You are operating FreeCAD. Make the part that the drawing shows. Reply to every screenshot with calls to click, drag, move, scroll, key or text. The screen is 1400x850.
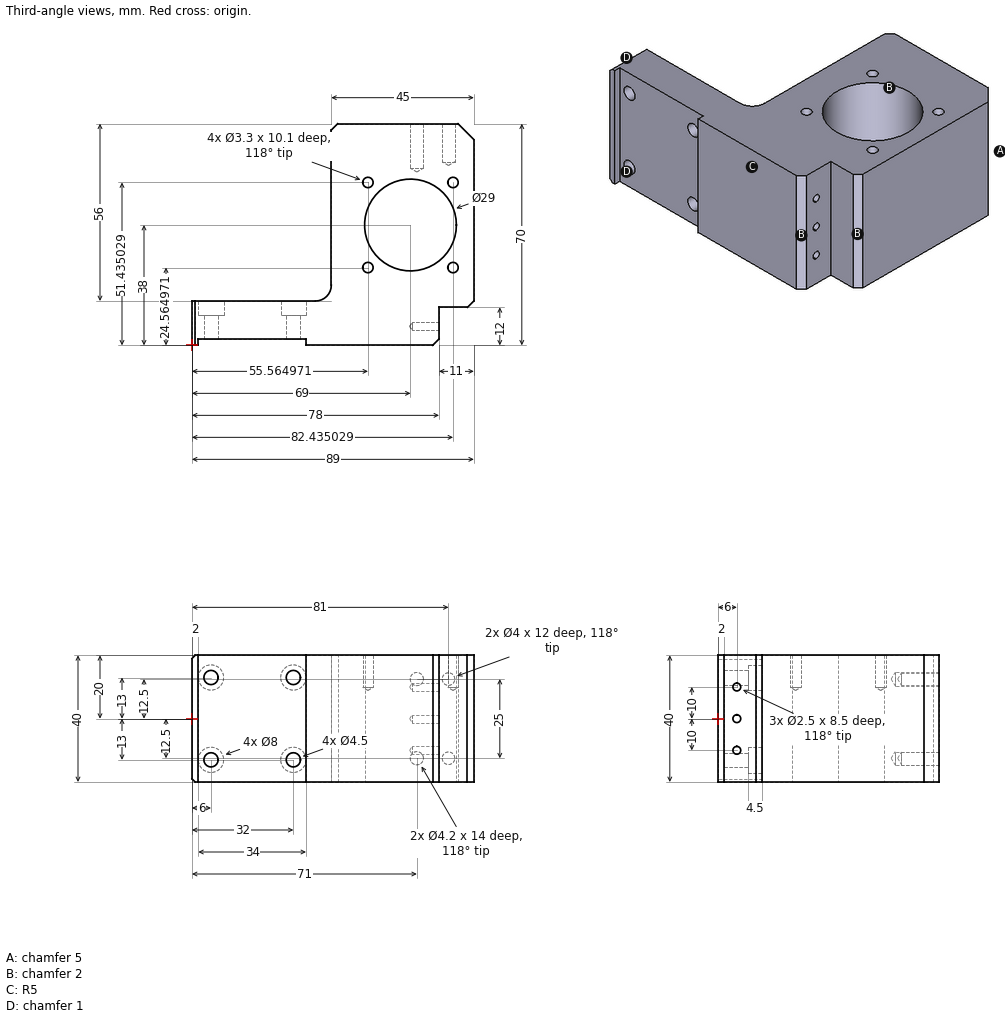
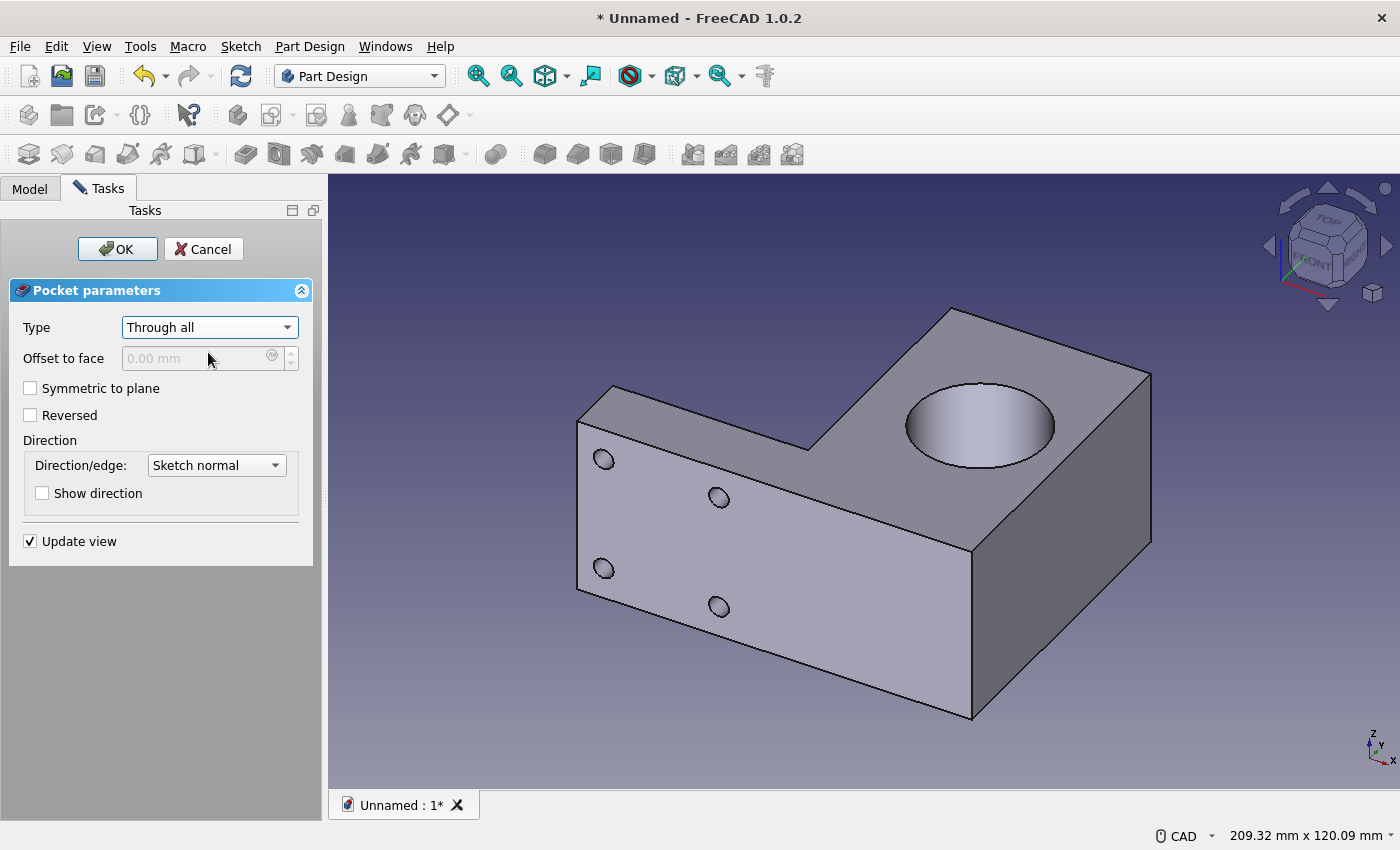
click(118, 249)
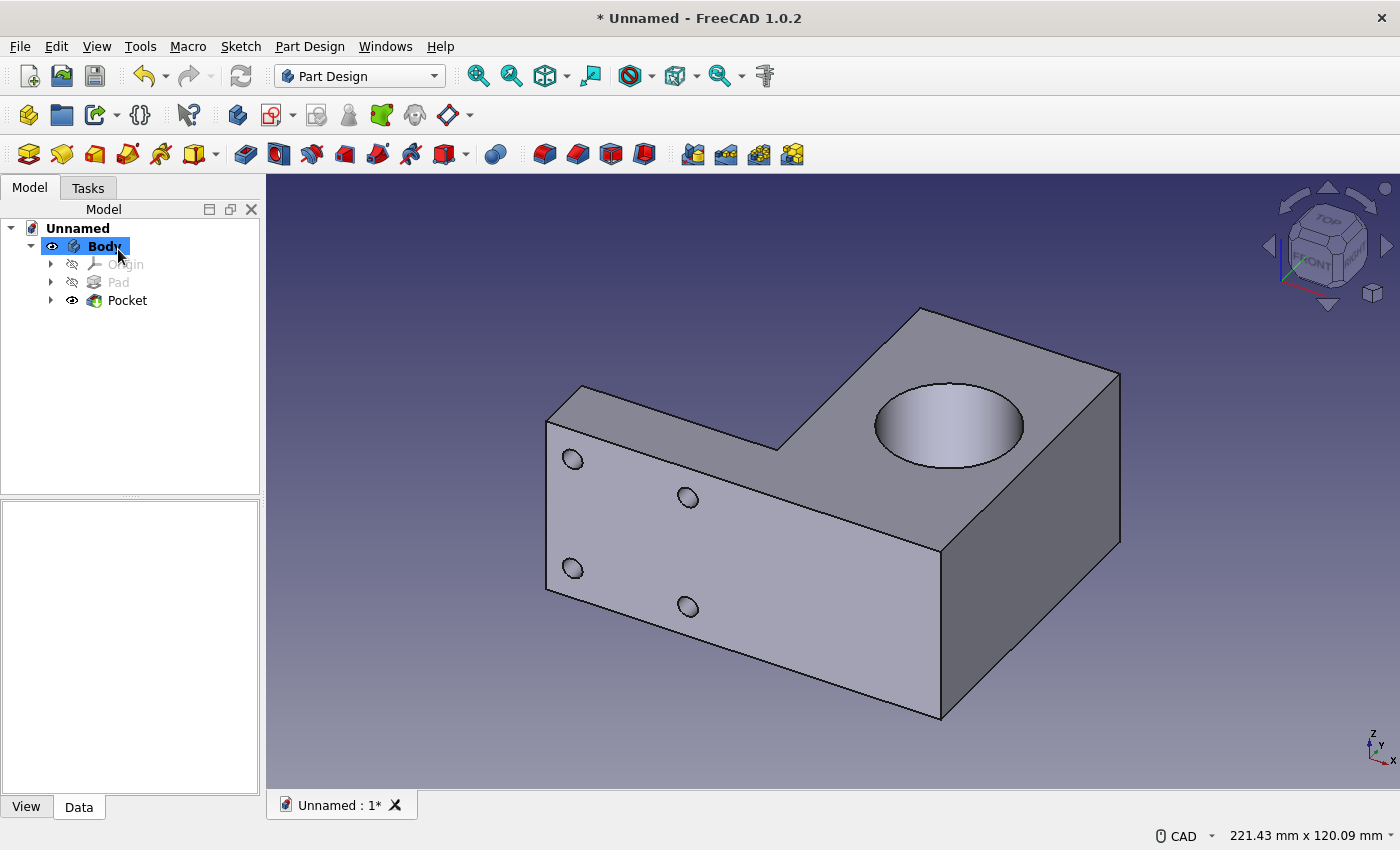
click(270, 116)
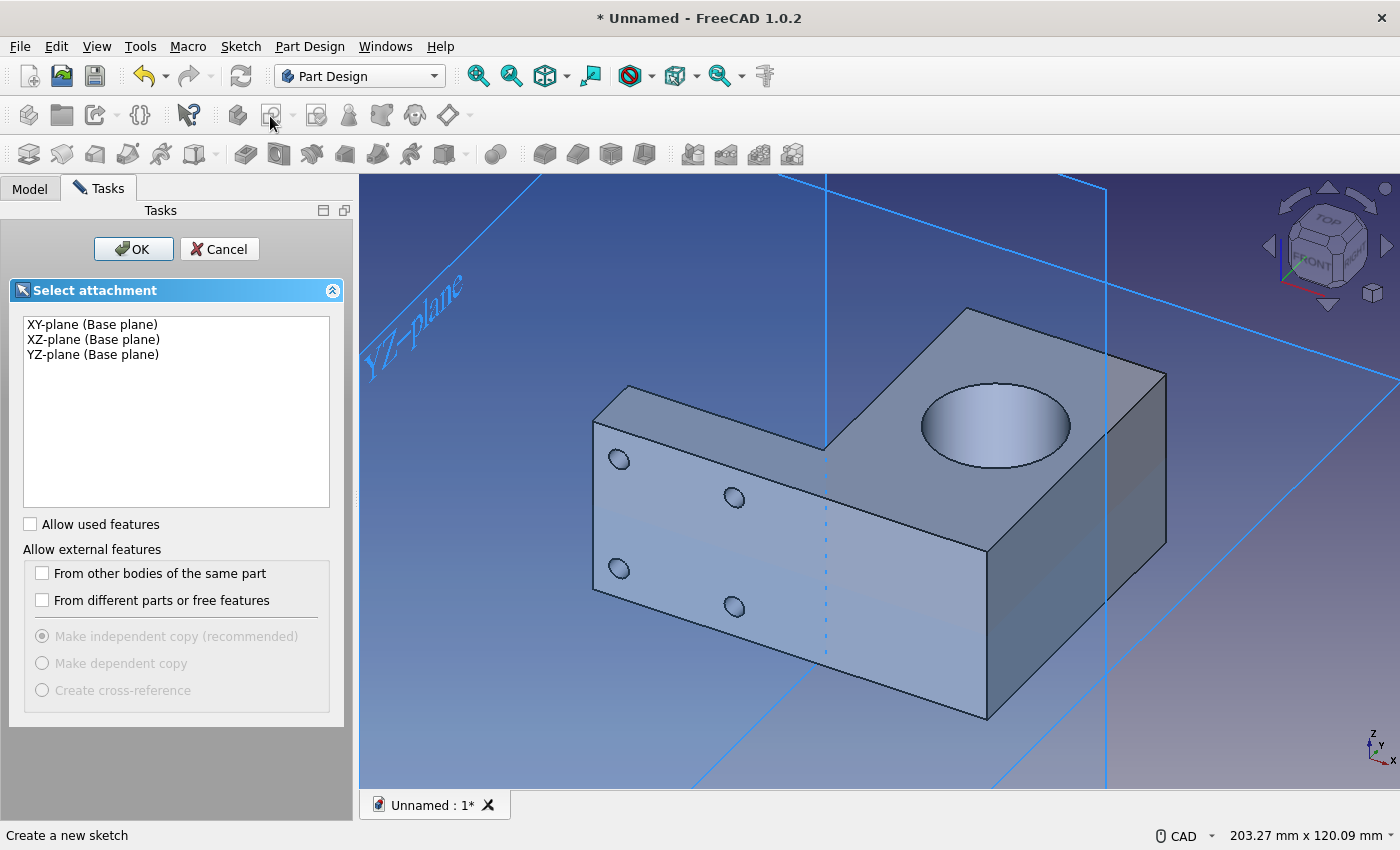
click(84, 340)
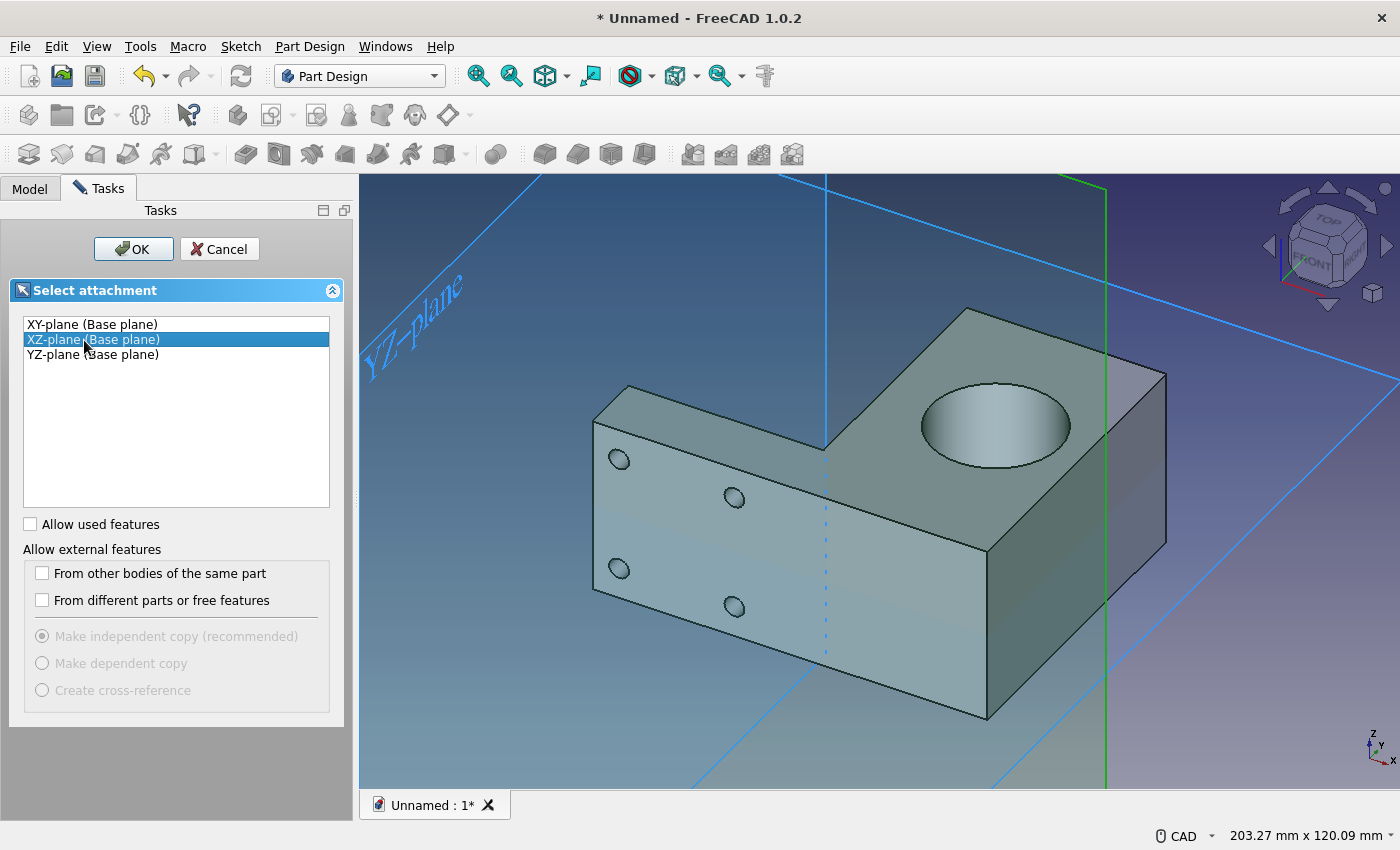
click(134, 249)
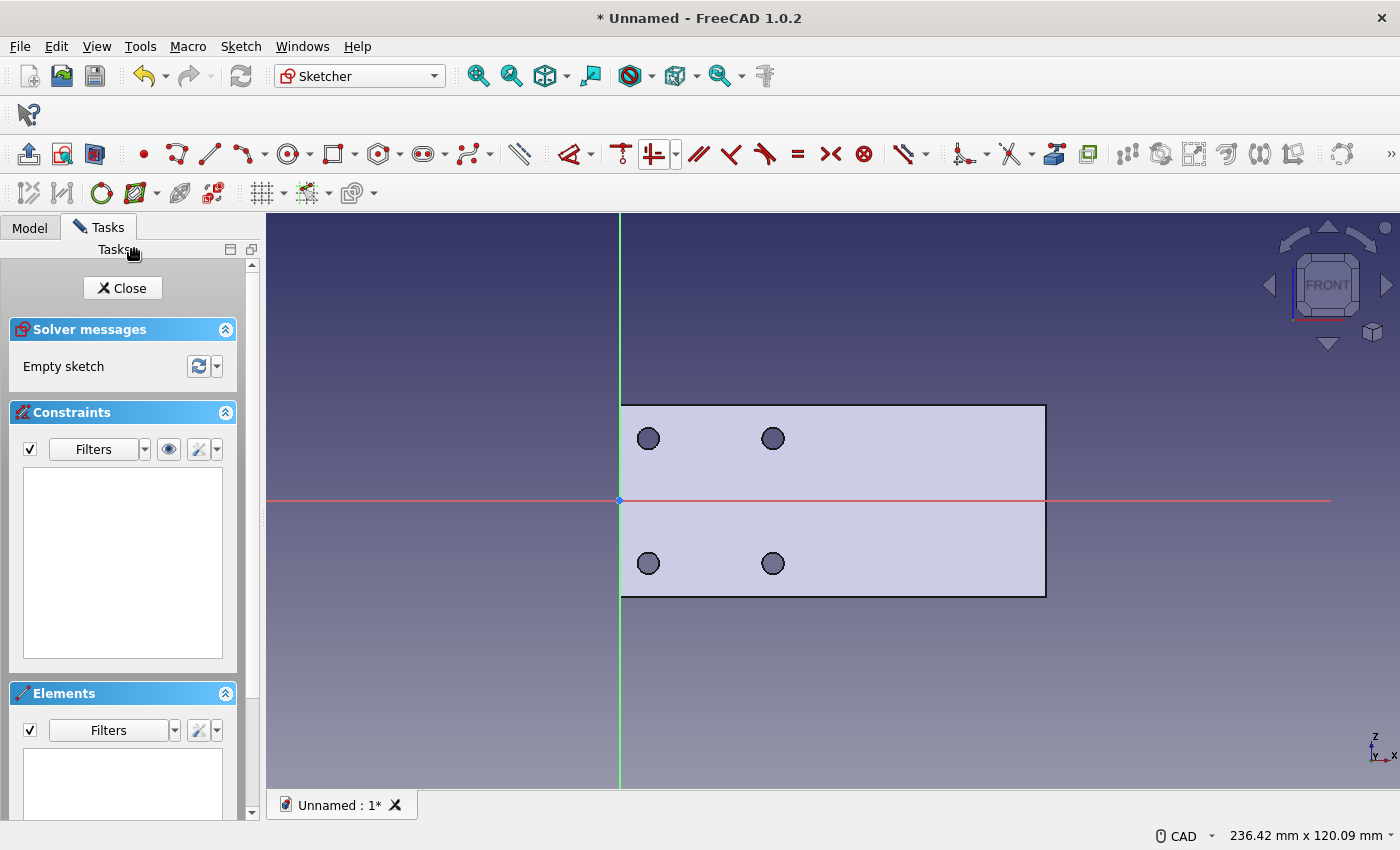
scroll(635, 501, up, 3)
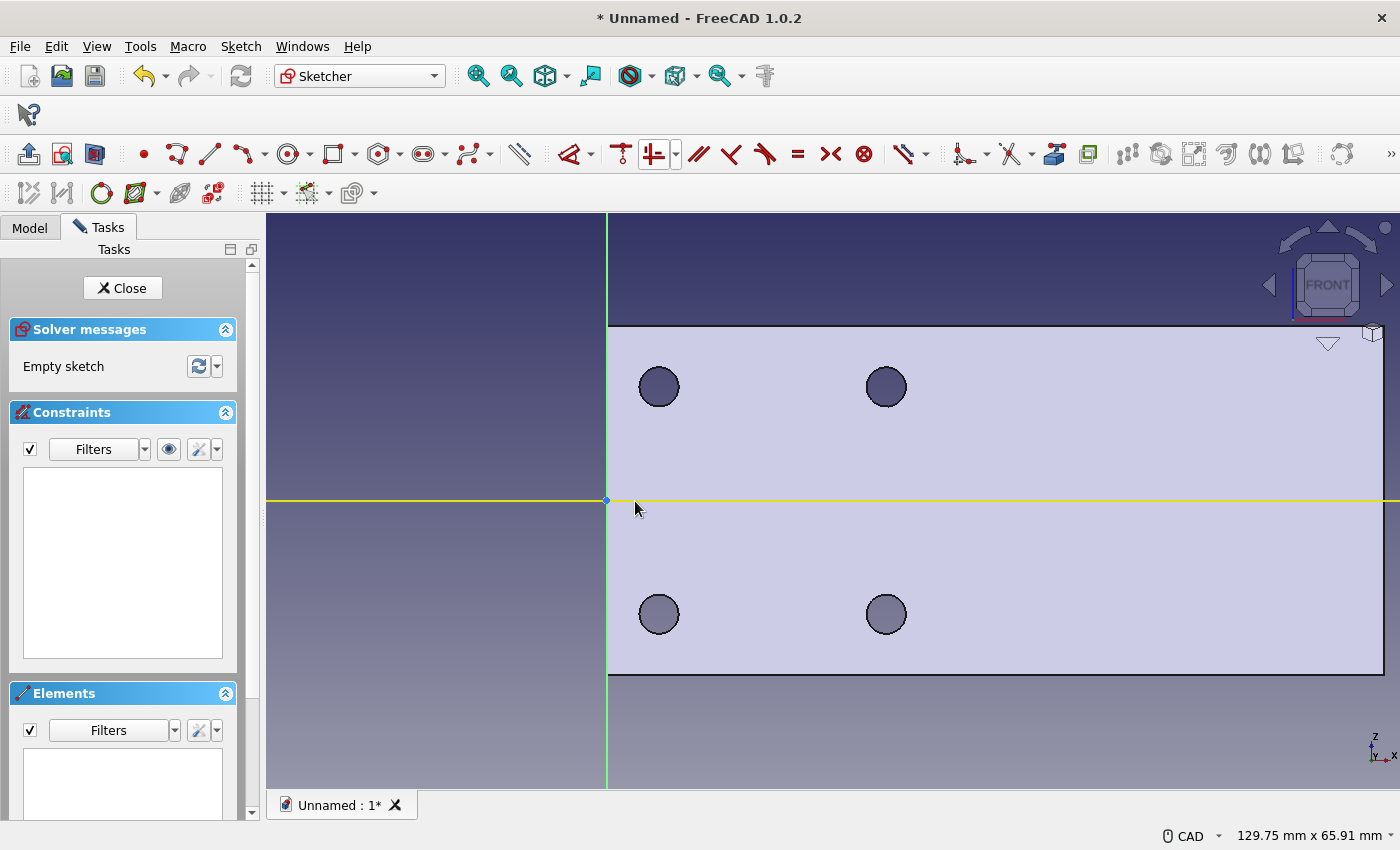
click(332, 154)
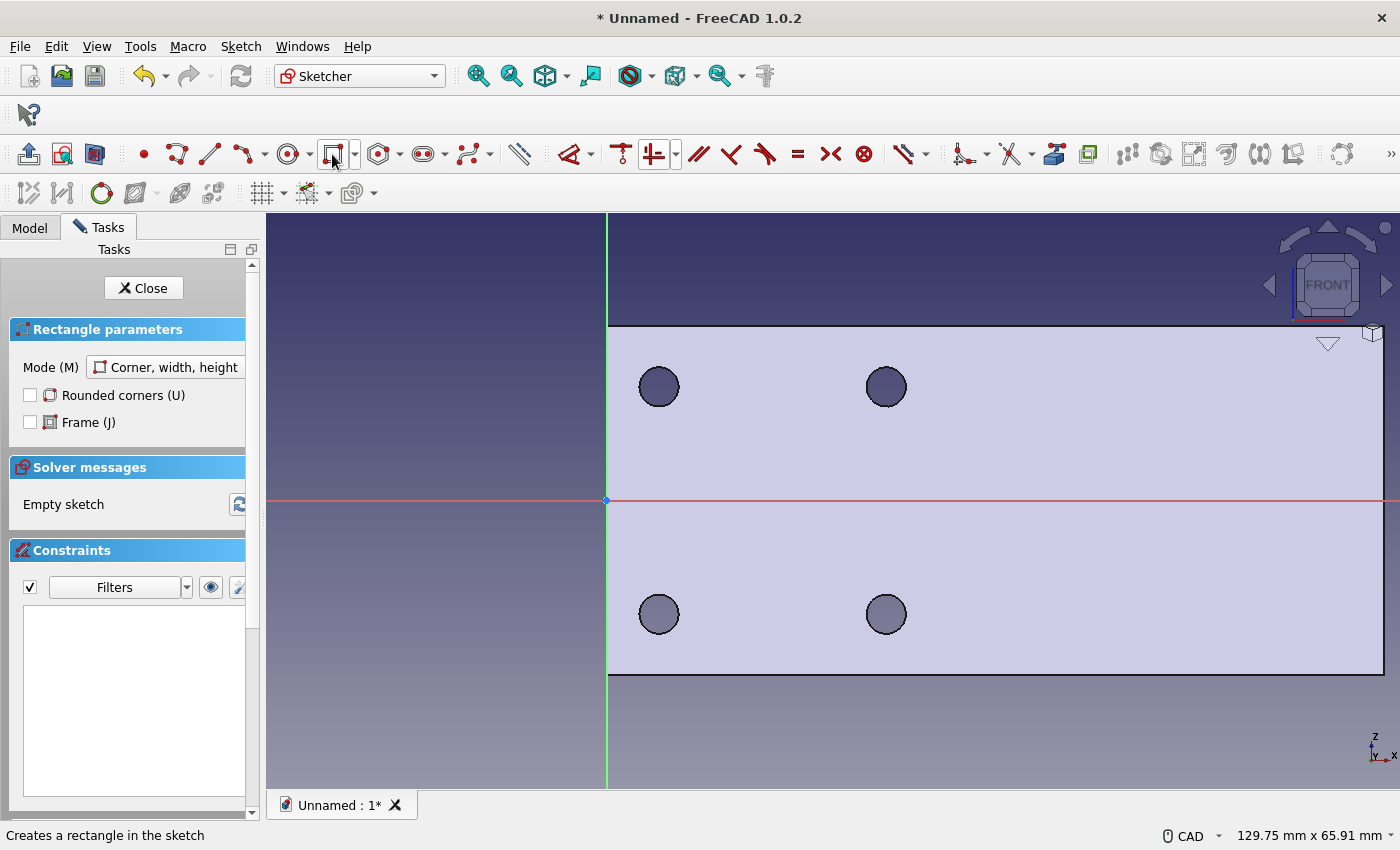
click(624, 326)
move(921, 675)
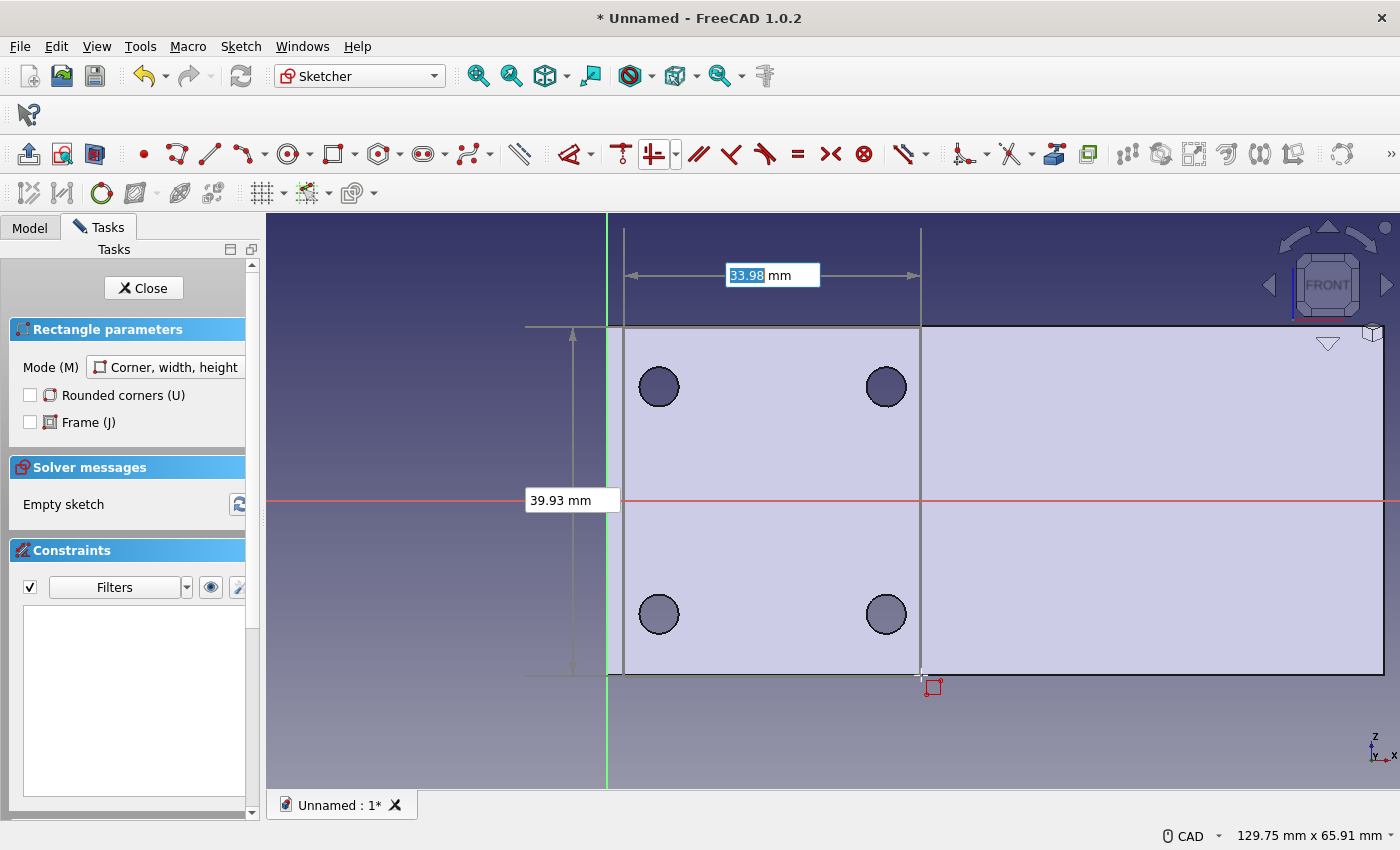
text(34)
key(Tab)
text(40)
key(Return)
key(Escape)